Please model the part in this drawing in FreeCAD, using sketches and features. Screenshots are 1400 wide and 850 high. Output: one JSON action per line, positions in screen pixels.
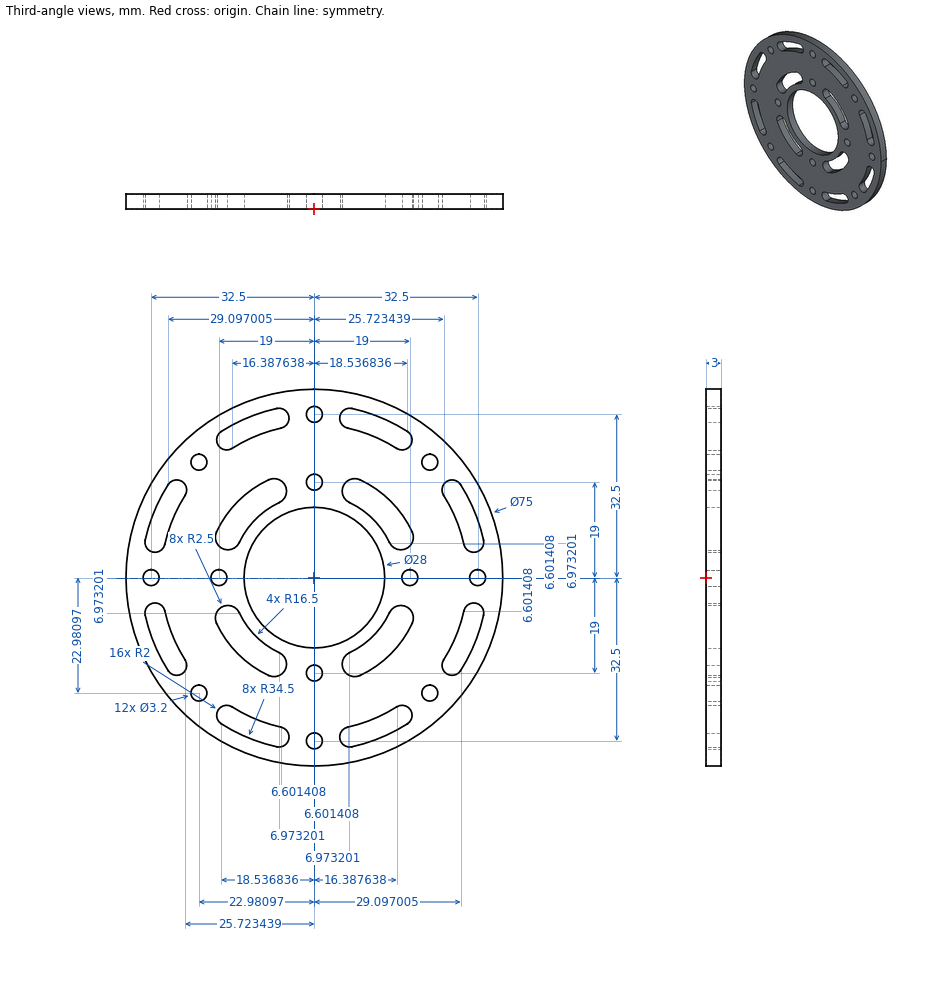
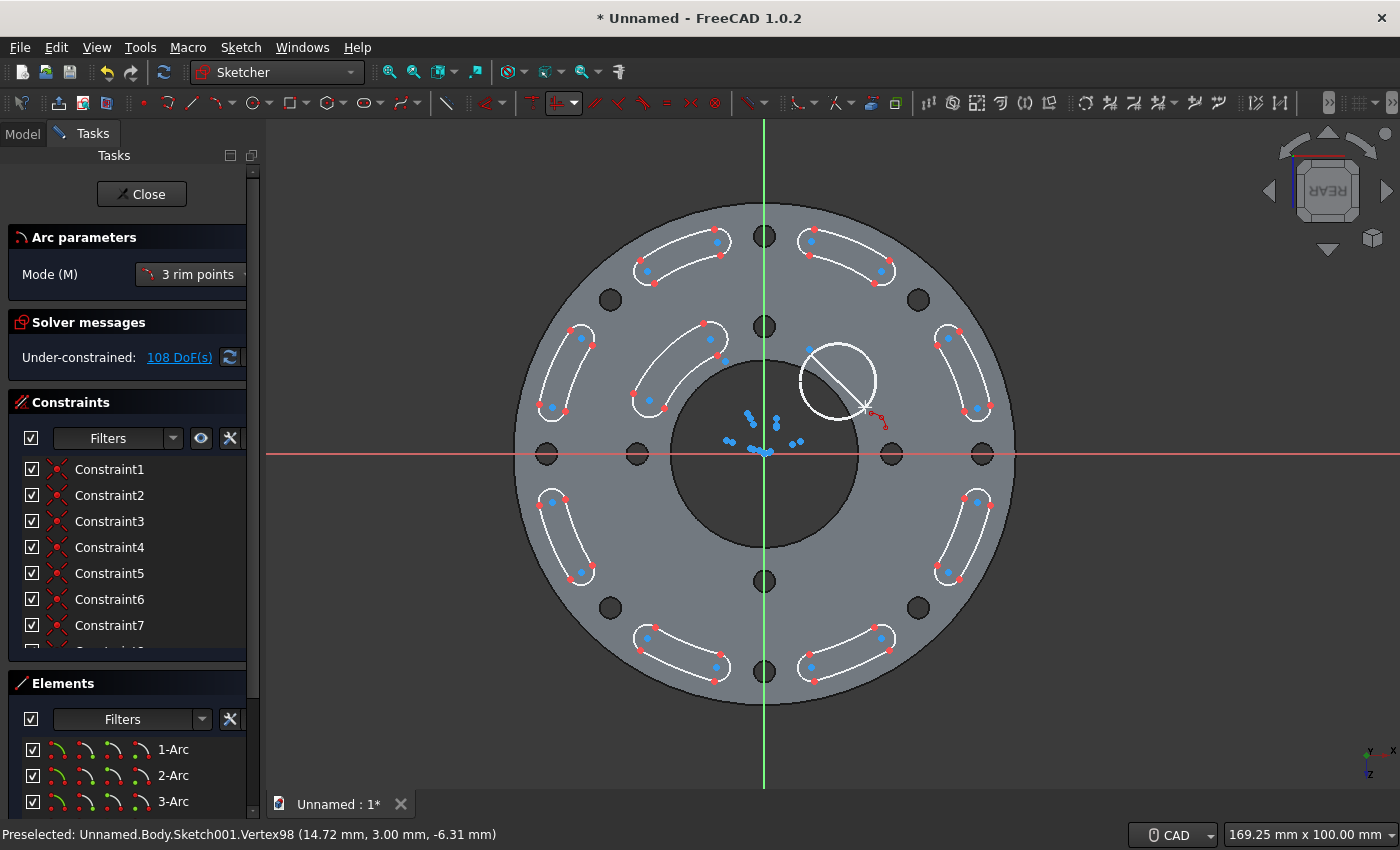
{"action": "scroll", "coordinate": [843, 376], "scroll_direction": "up", "scroll_amount": 5}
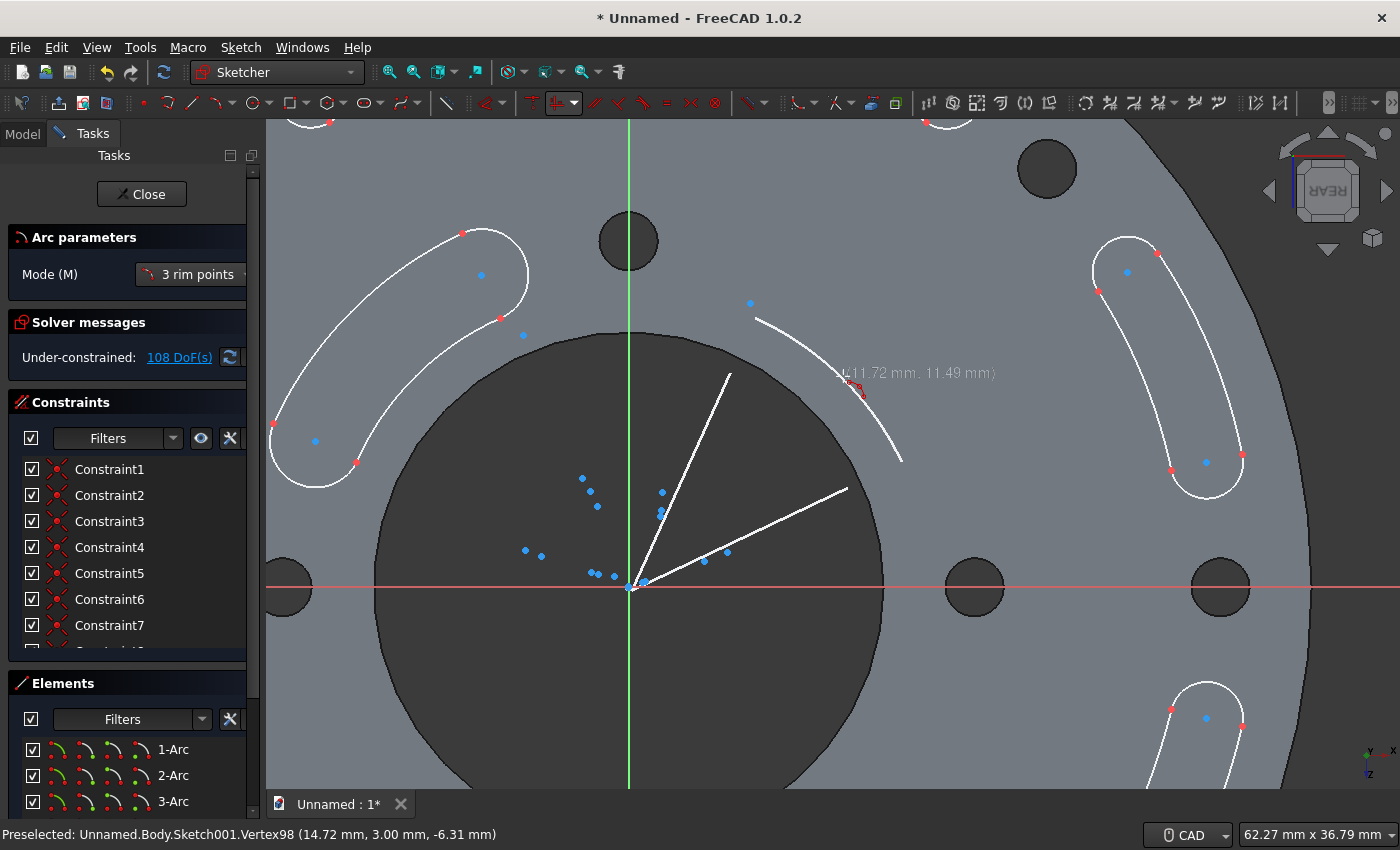
{"action": "left_click", "coordinate": [841, 375]}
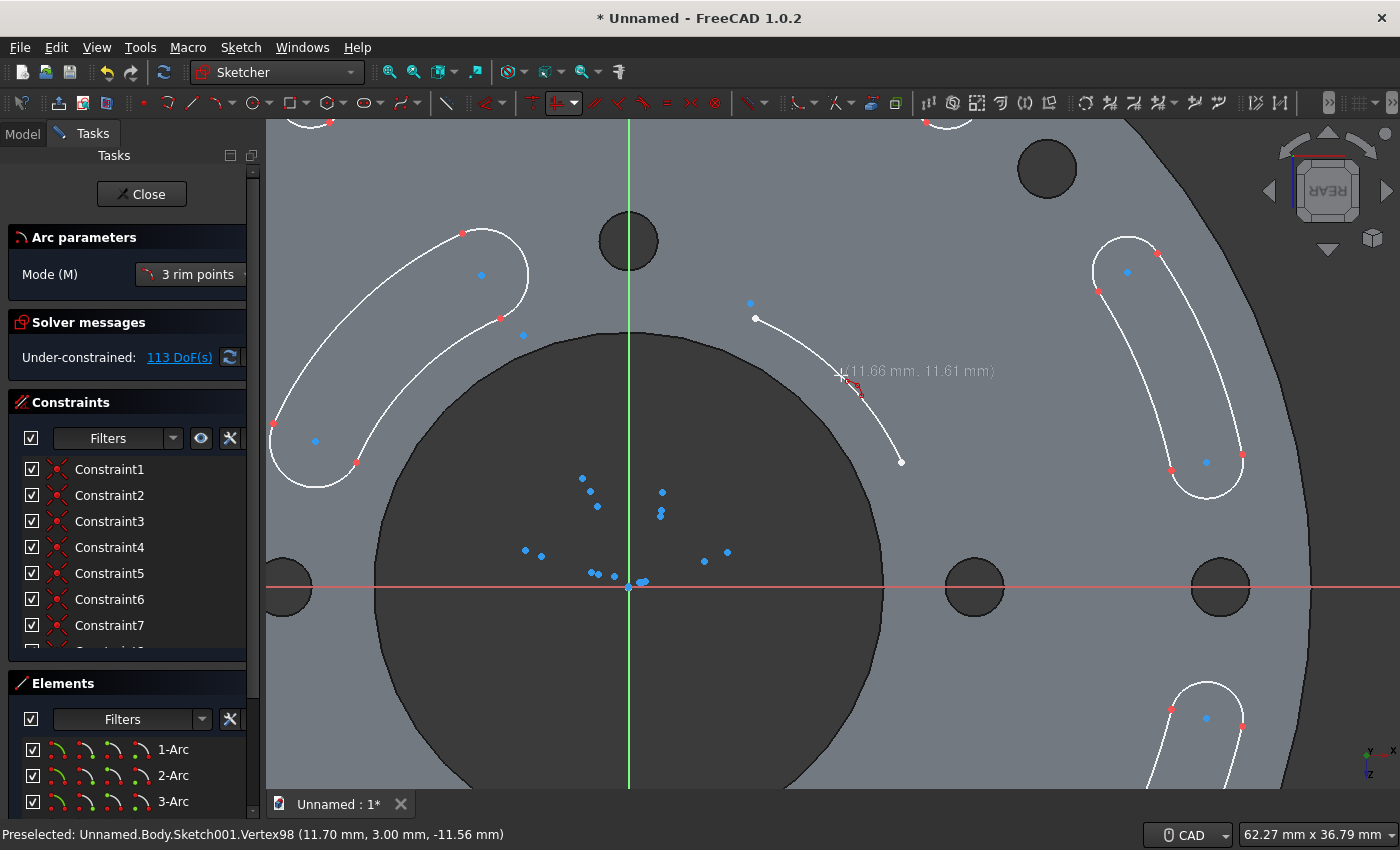
{"action": "left_click", "coordinate": [902, 462]}
{"action": "left_click", "coordinate": [984, 422]}
{"action": "left_click", "coordinate": [962, 482]}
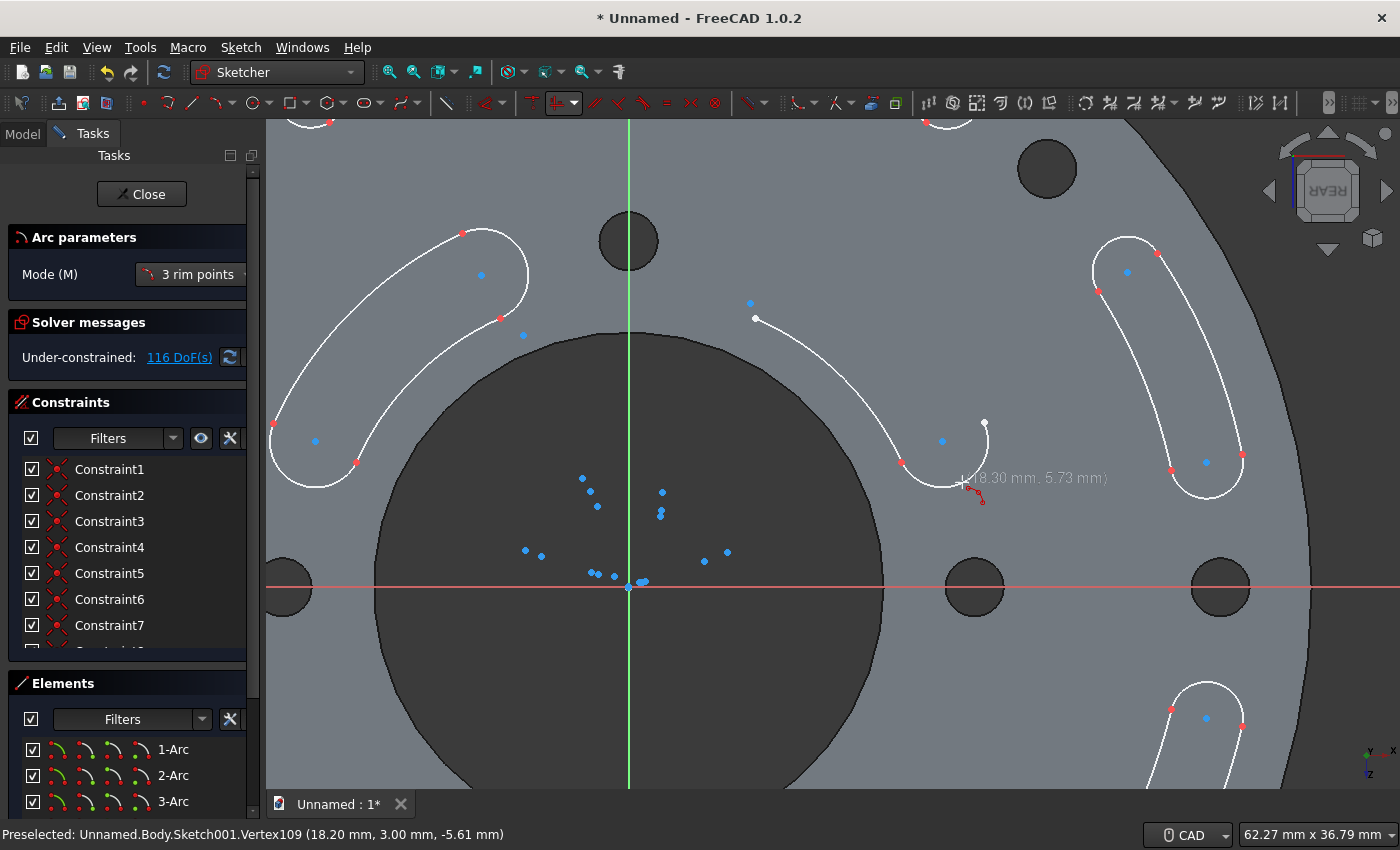
{"action": "left_click", "coordinate": [984, 423]}
{"action": "left_click", "coordinate": [794, 232]}
{"action": "left_click", "coordinate": [906, 310]}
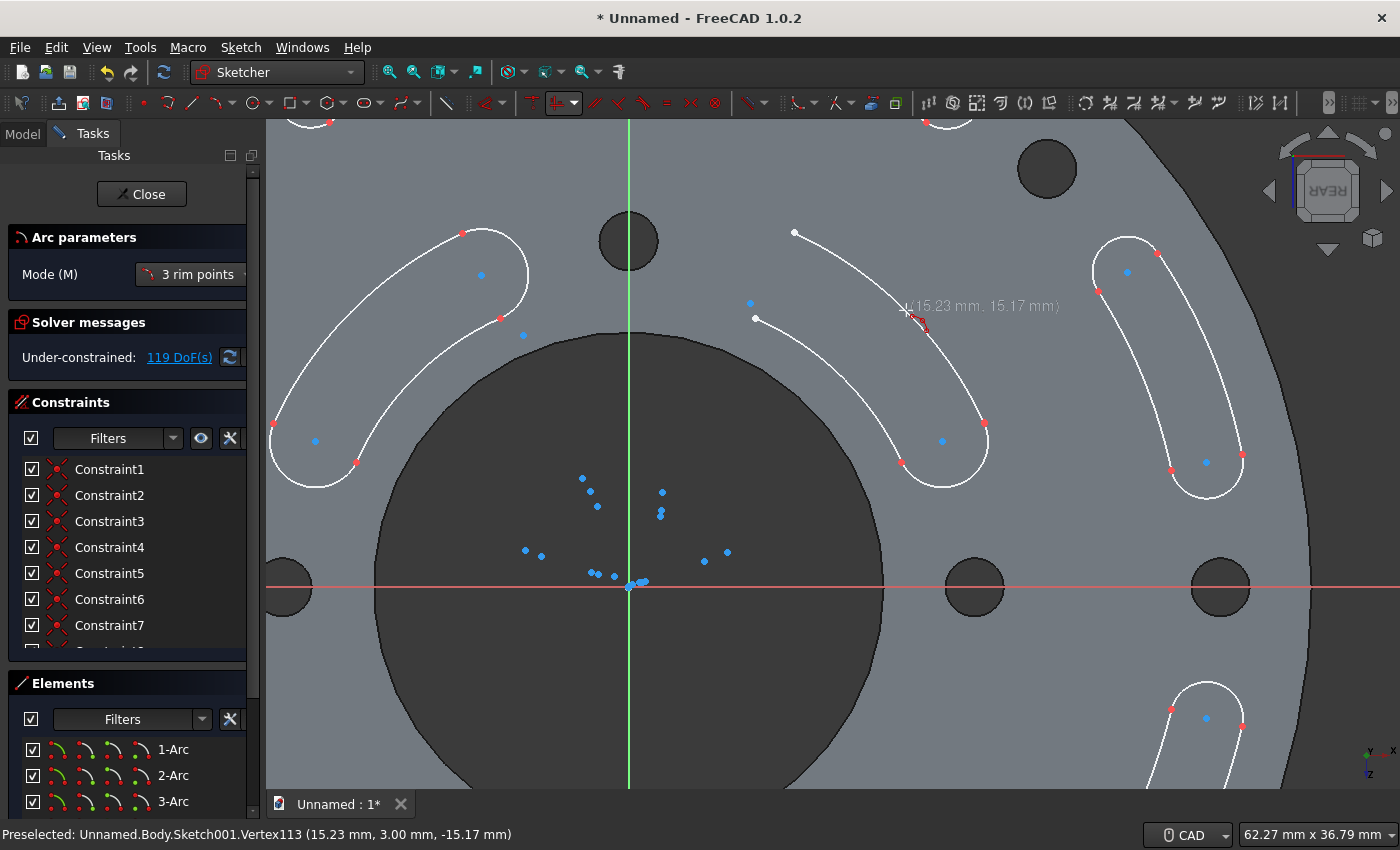
{"action": "left_click", "coordinate": [794, 233]}
{"action": "left_click", "coordinate": [755, 318]}
{"action": "left_click", "coordinate": [734, 255]}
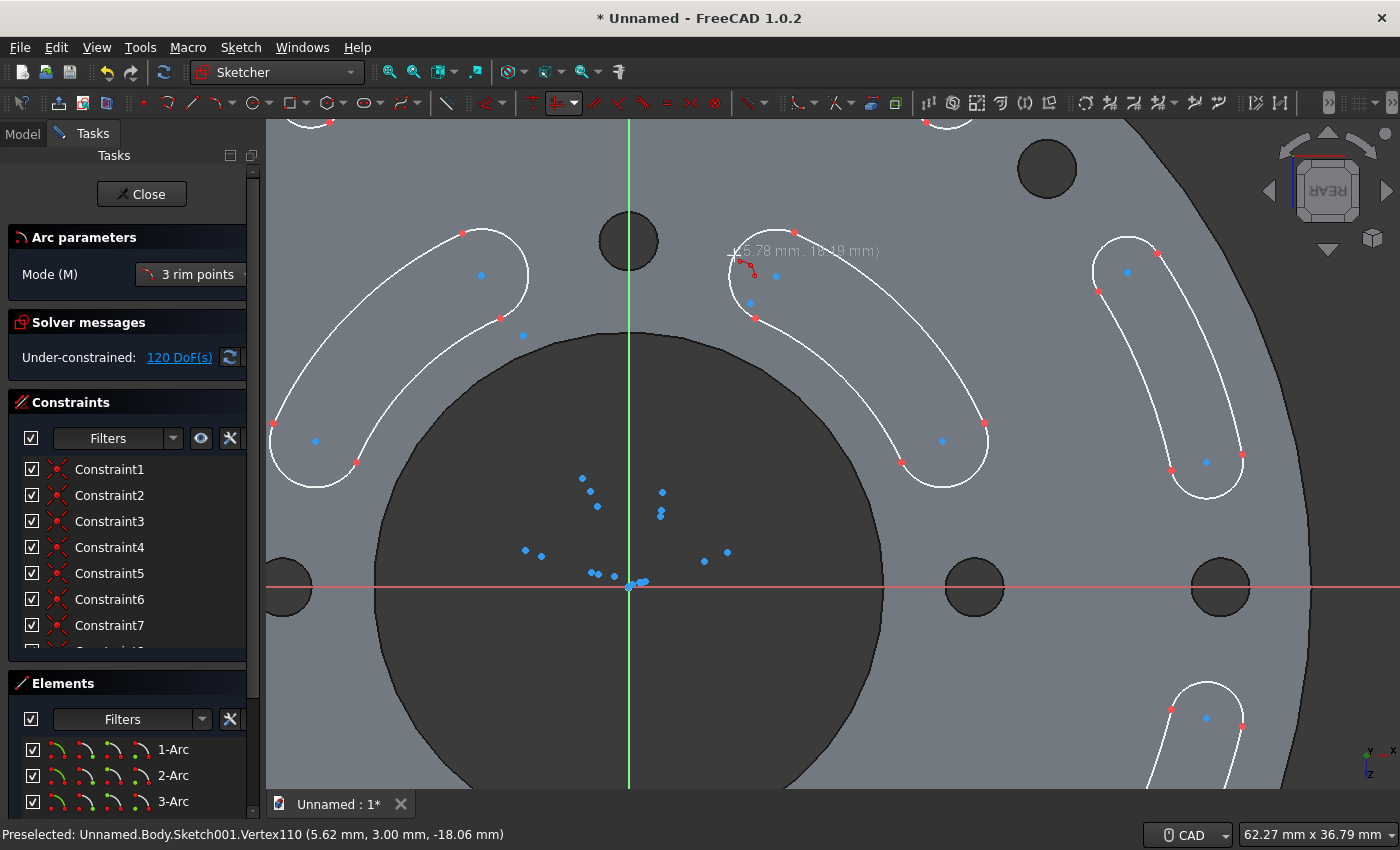
{"action": "left_click", "coordinate": [901, 714]}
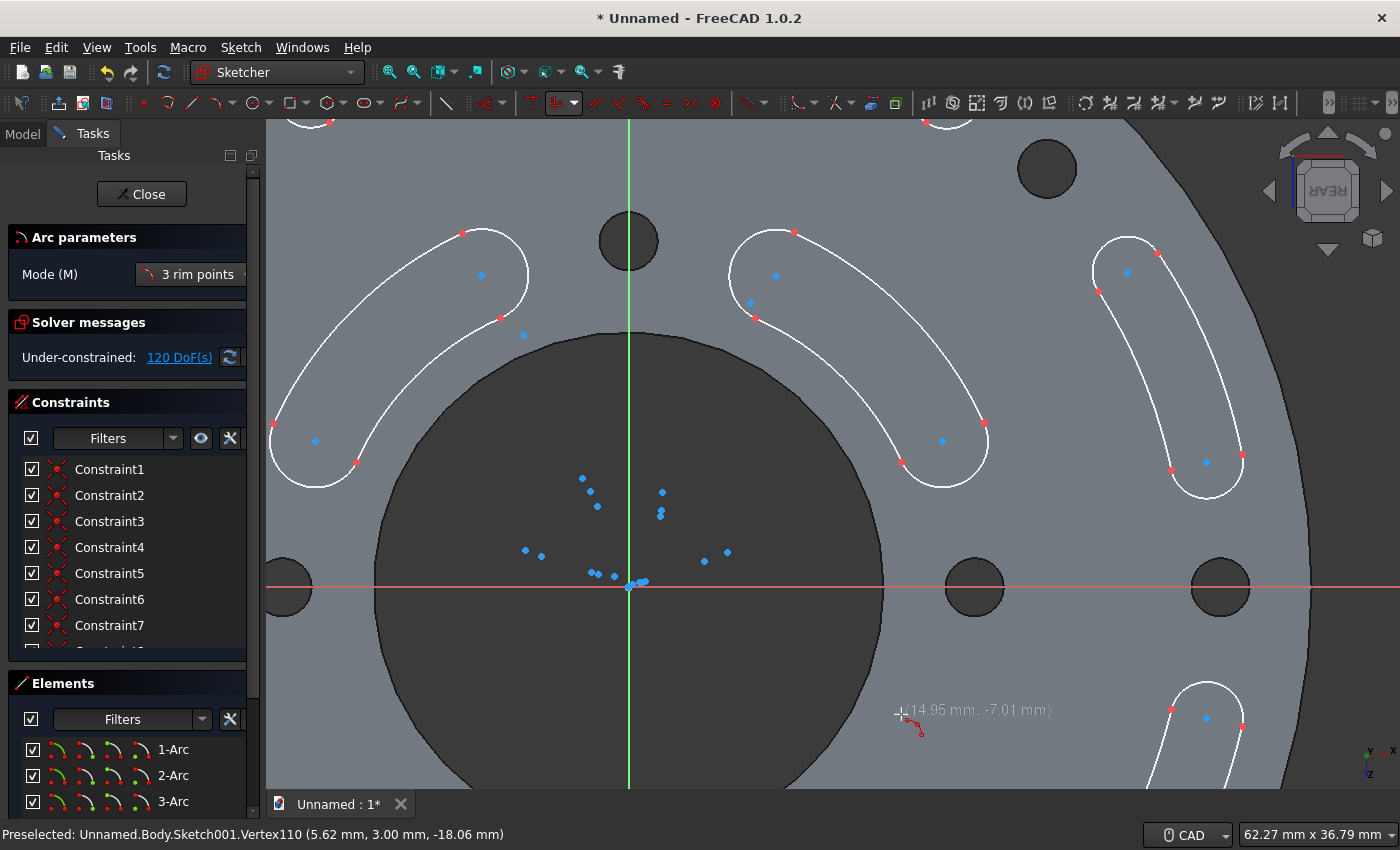
{"action": "scroll", "coordinate": [844, 376], "scroll_direction": "down", "scroll_amount": 5}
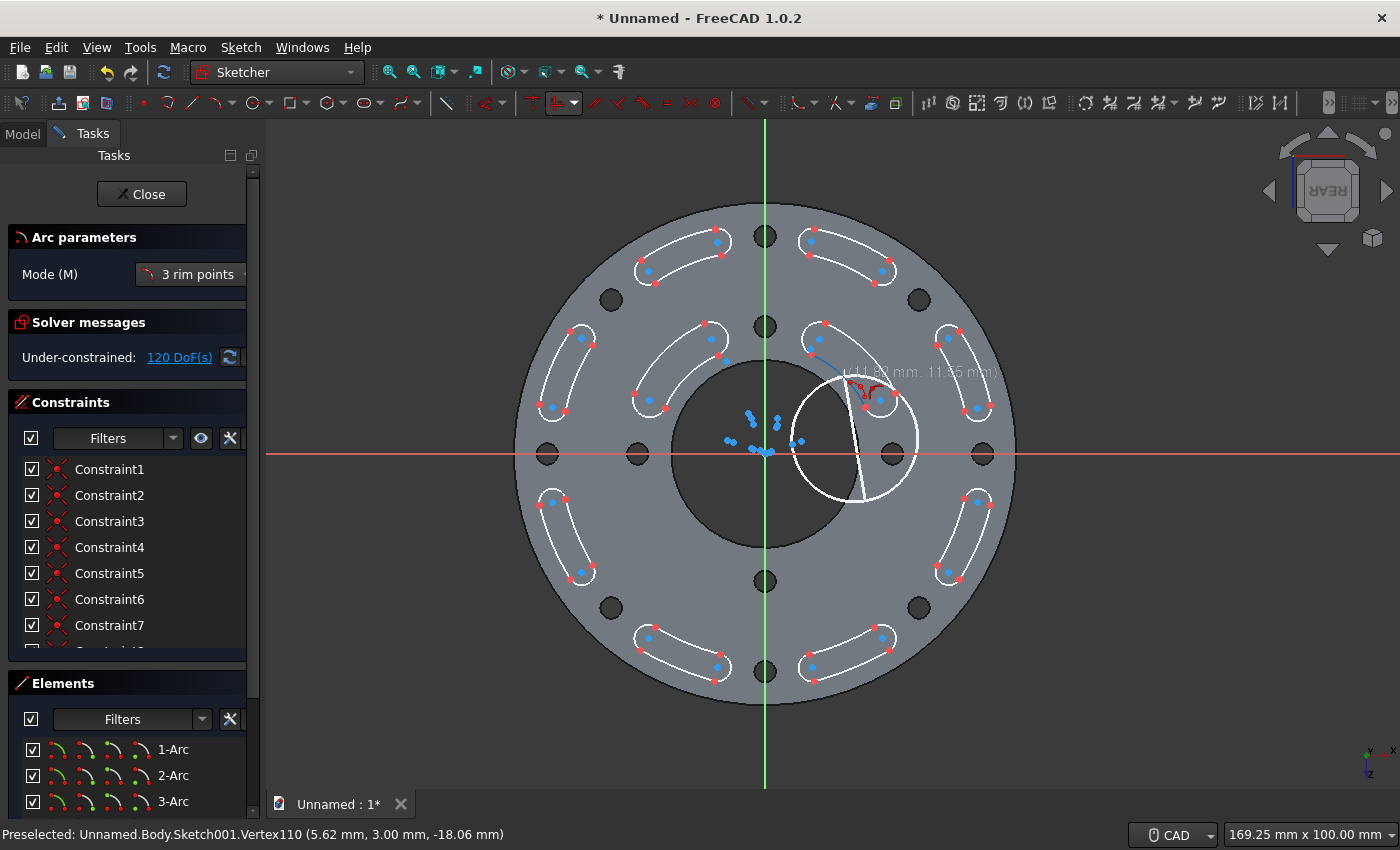
{"action": "left_click", "coordinate": [812, 554]}